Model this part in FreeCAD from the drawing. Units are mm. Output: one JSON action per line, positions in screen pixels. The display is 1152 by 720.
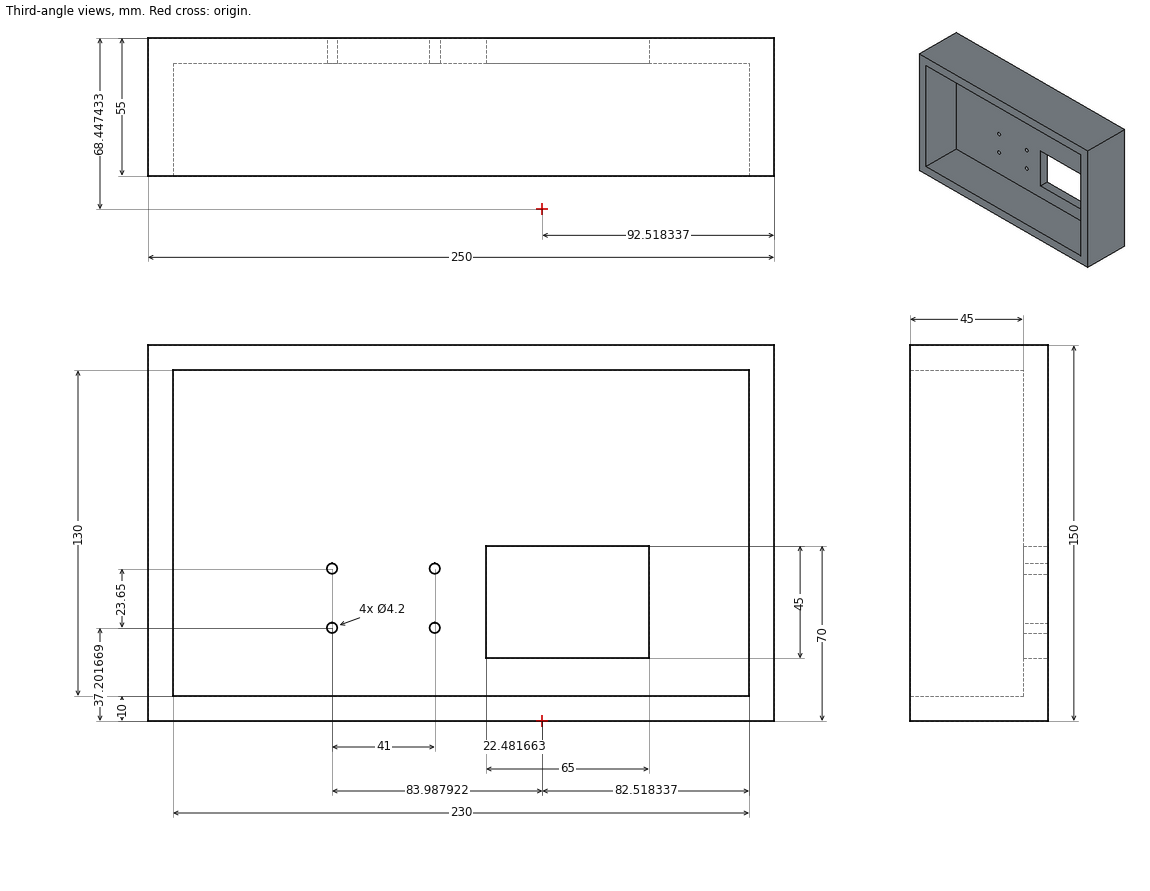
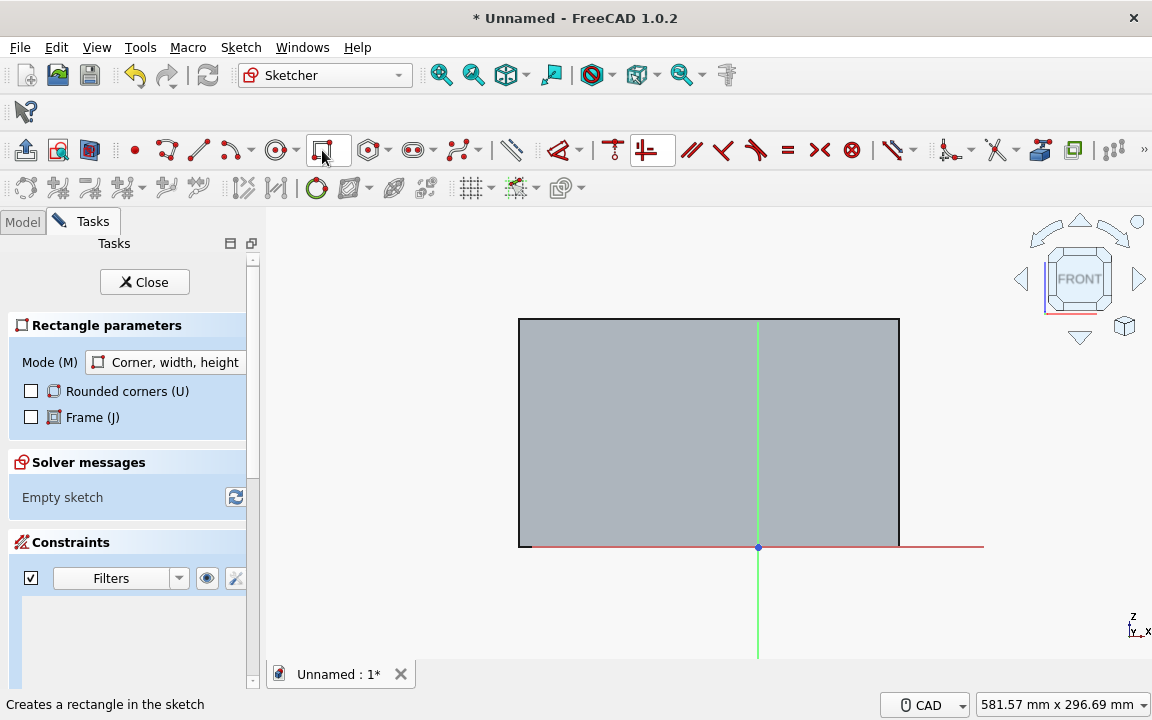
{"action": "left_click", "coordinate": [534, 334]}
{"action": "left_click", "coordinate": [884, 532]}
{"action": "key", "text": "Escape"}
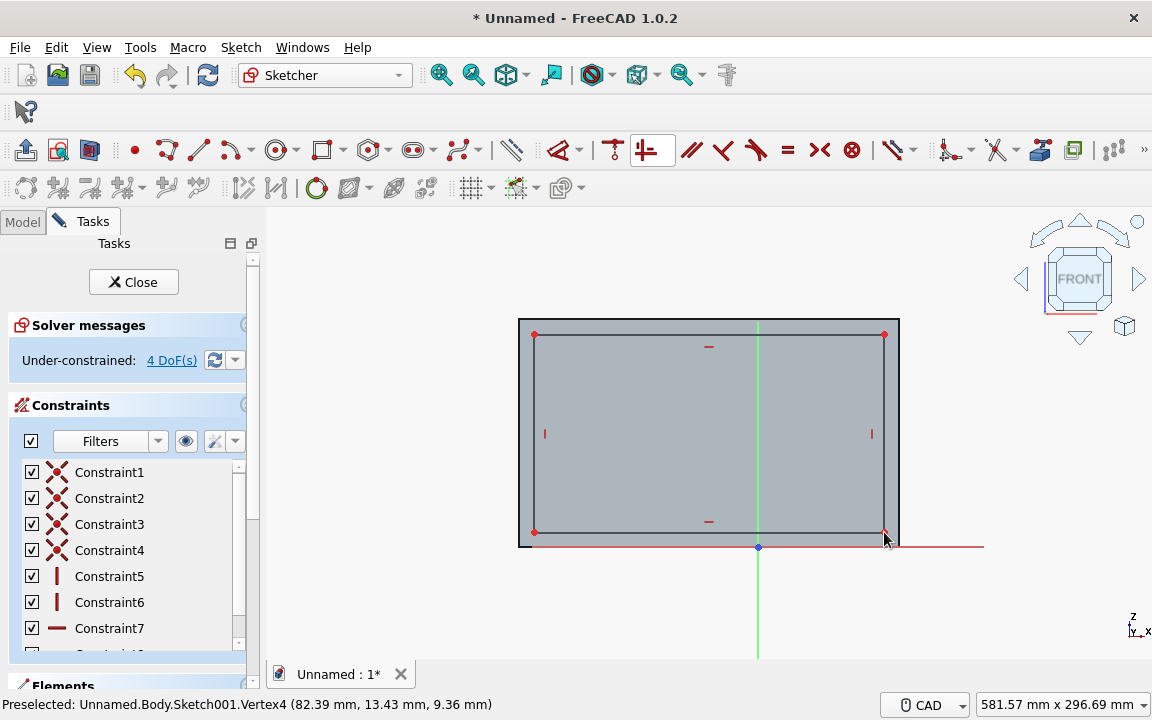
{"action": "left_click", "coordinate": [558, 150]}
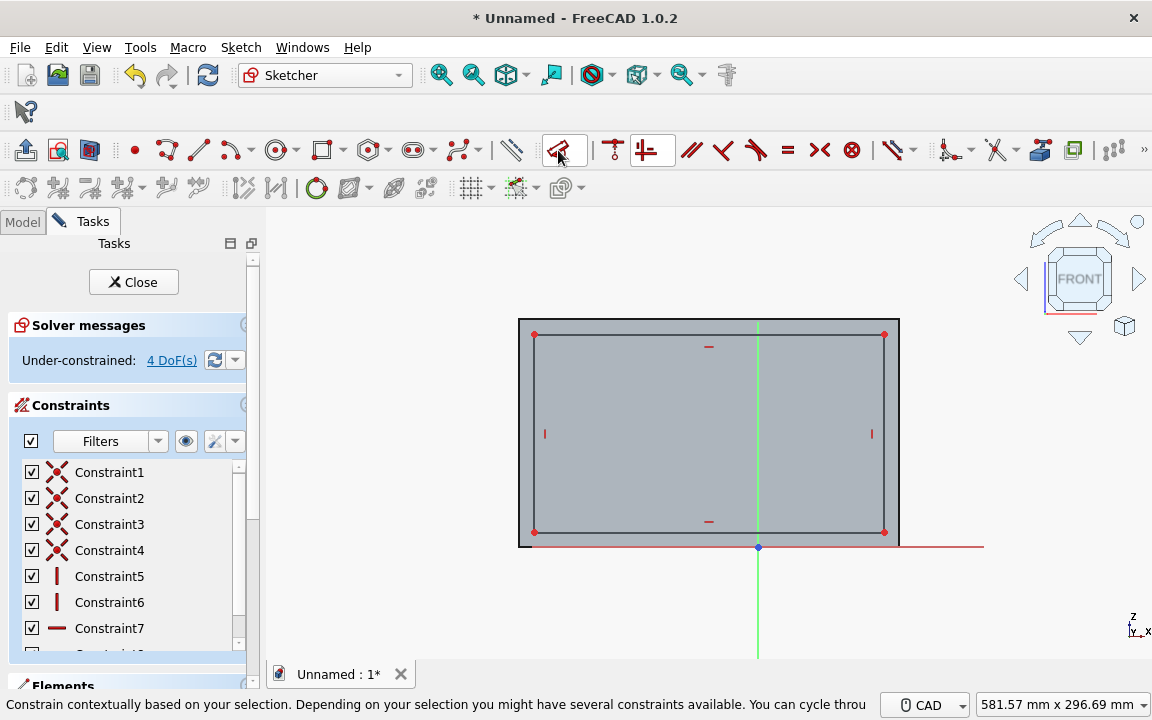
{"action": "left_click", "coordinate": [534, 394]}
{"action": "left_click", "coordinate": [500, 434]}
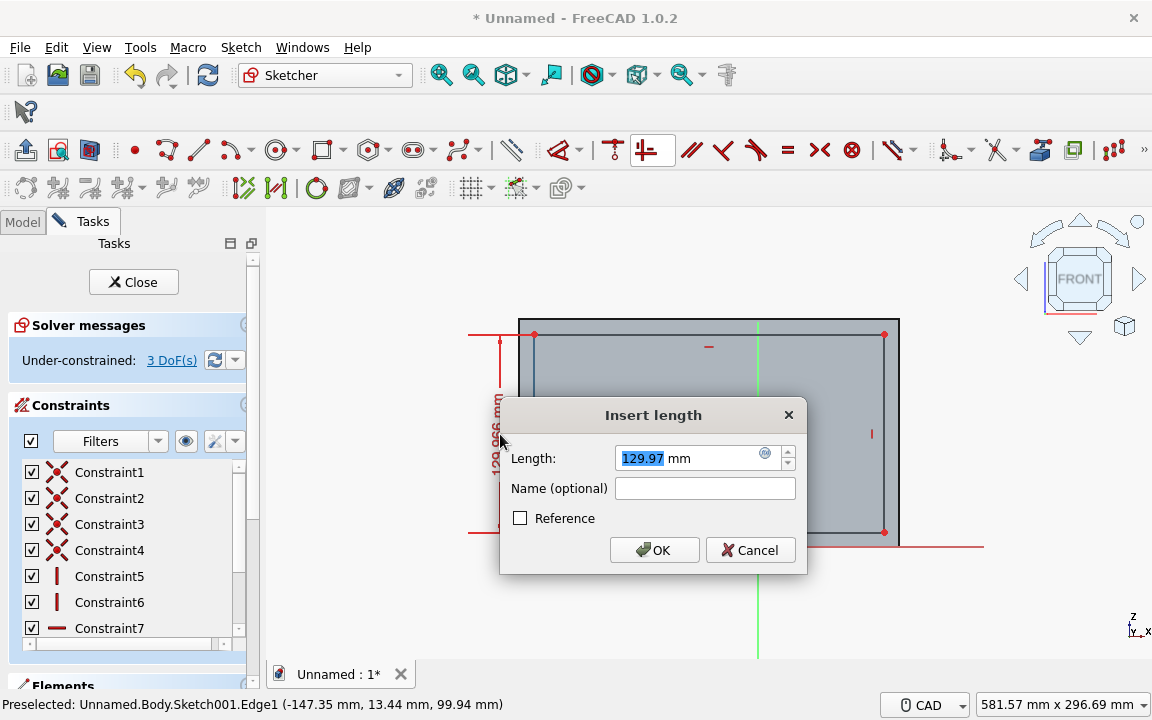
{"action": "type", "text": "130"}
{"action": "key", "text": "Return"}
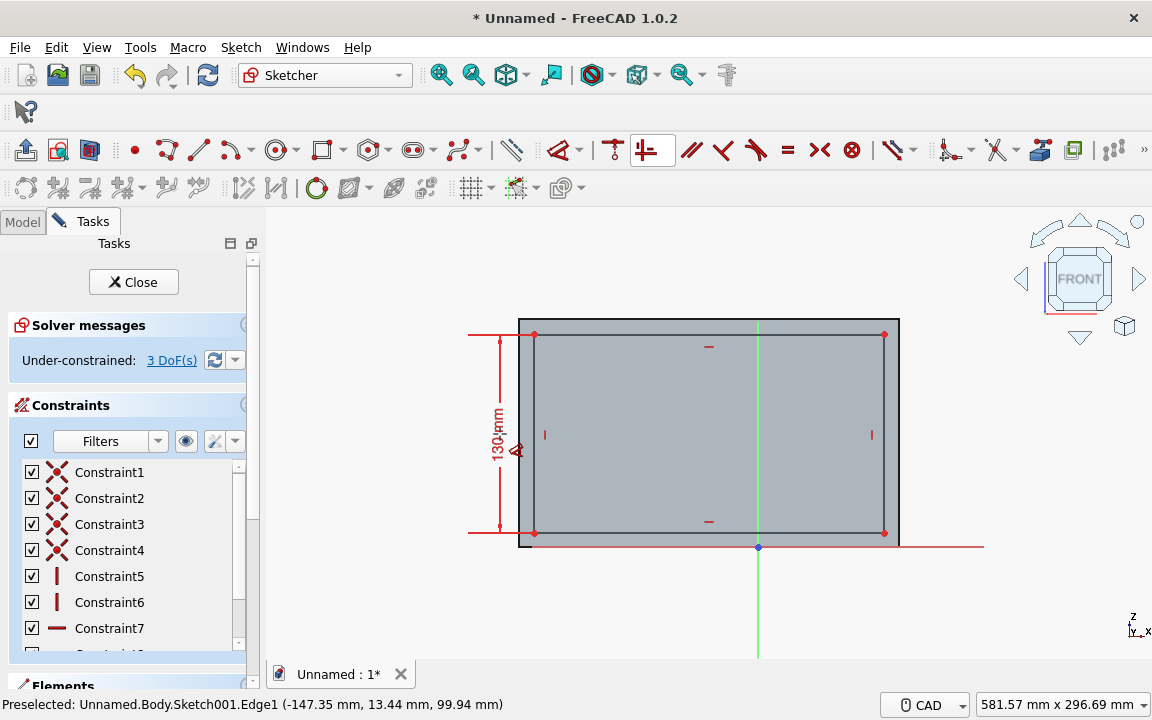
{"action": "left_click", "coordinate": [639, 533]}
{"action": "left_click", "coordinate": [709, 567]}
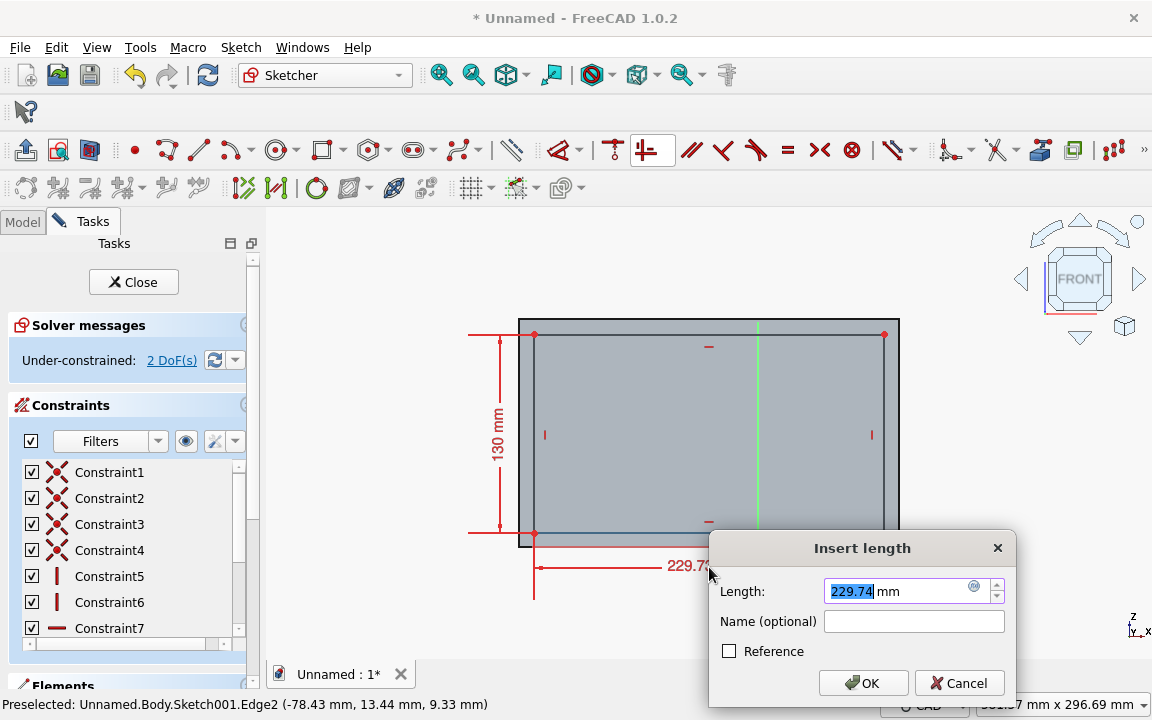
{"action": "type", "text": "230"}
{"action": "key", "text": "Return"}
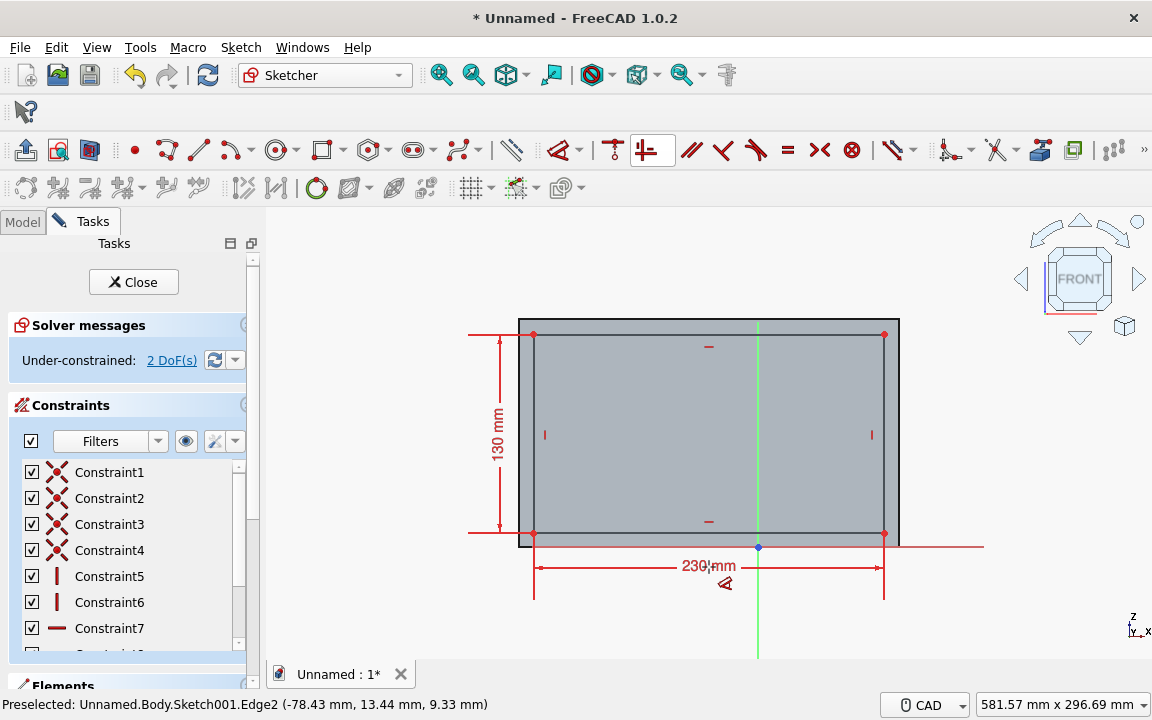
{"action": "scroll", "coordinate": [534, 533], "scroll_direction": "up", "scroll_amount": 5}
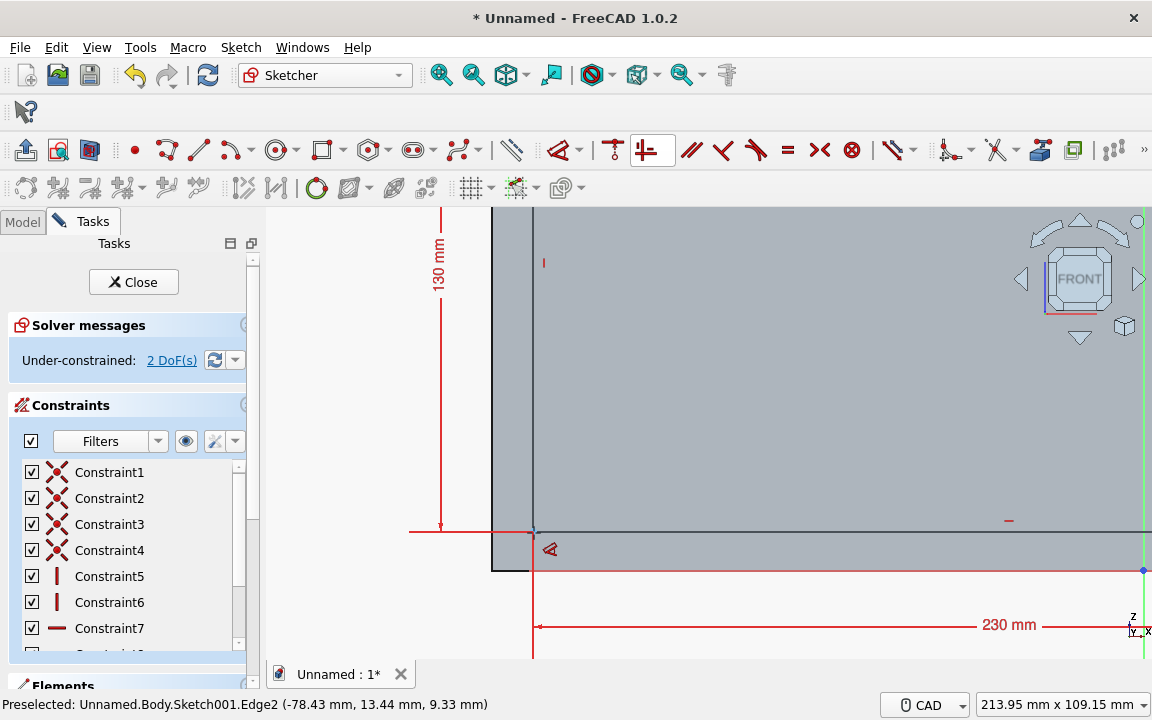
{"action": "left_click", "coordinate": [533, 532]}
{"action": "left_click", "coordinate": [499, 551]}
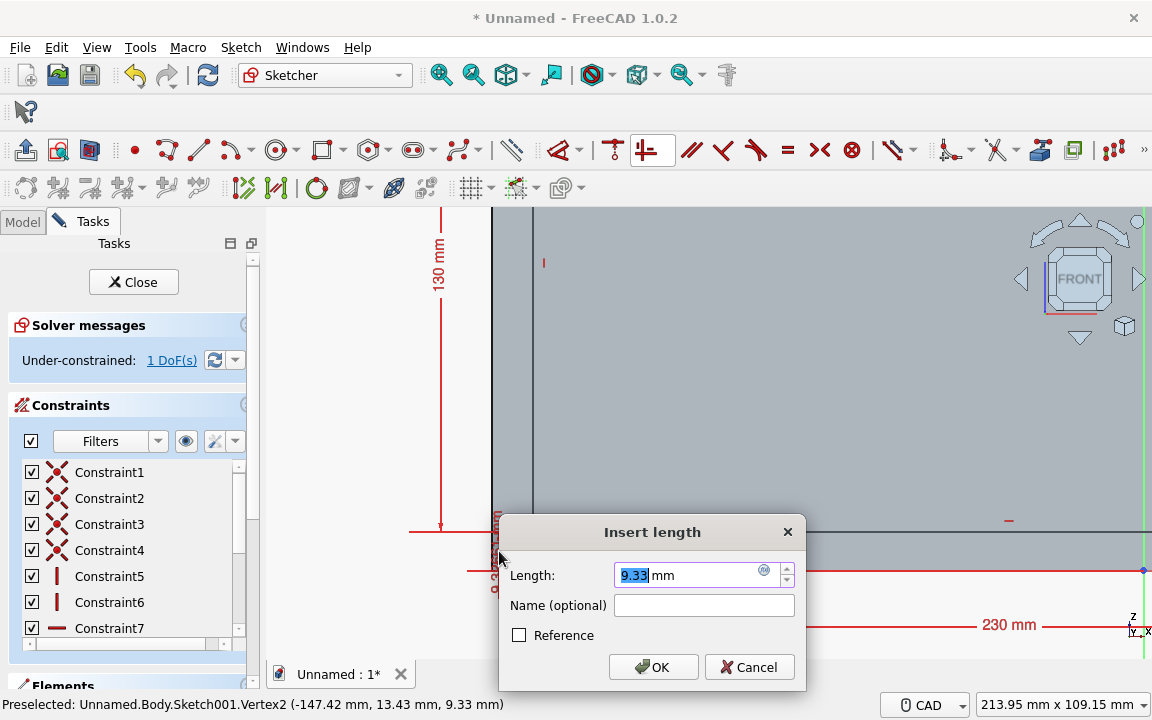
{"action": "type", "text": "10"}
{"action": "key", "text": "Return"}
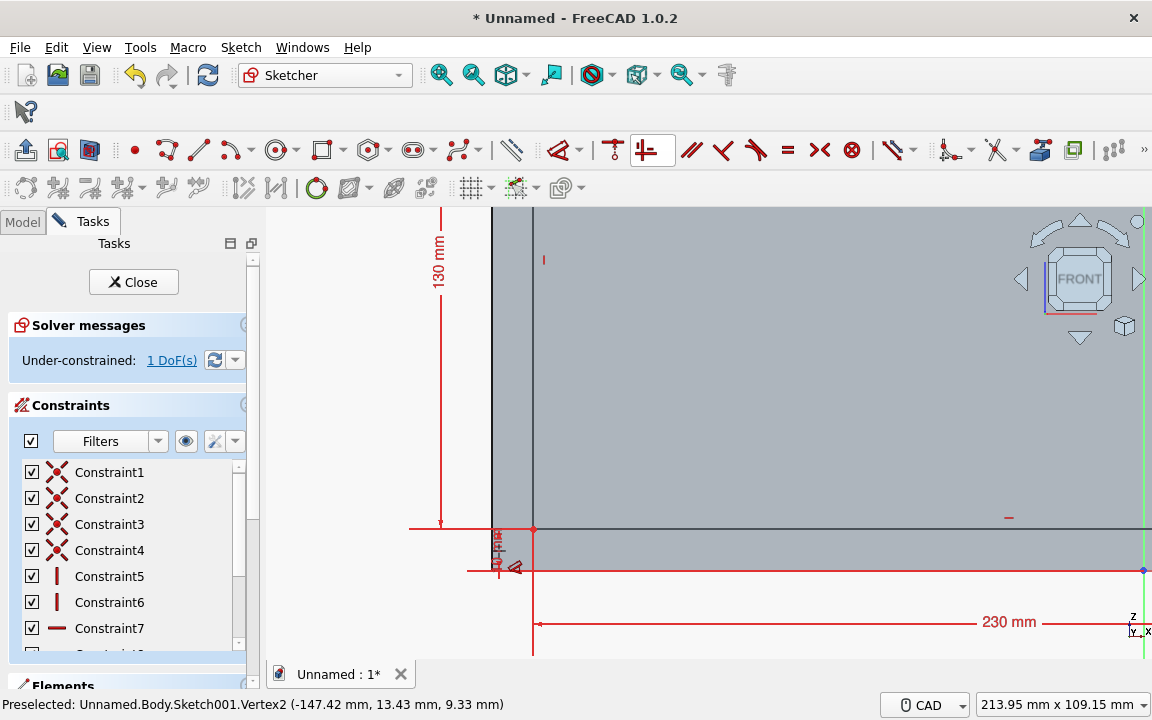
{"action": "scroll", "coordinate": [340, 557], "scroll_direction": "down", "scroll_amount": 4}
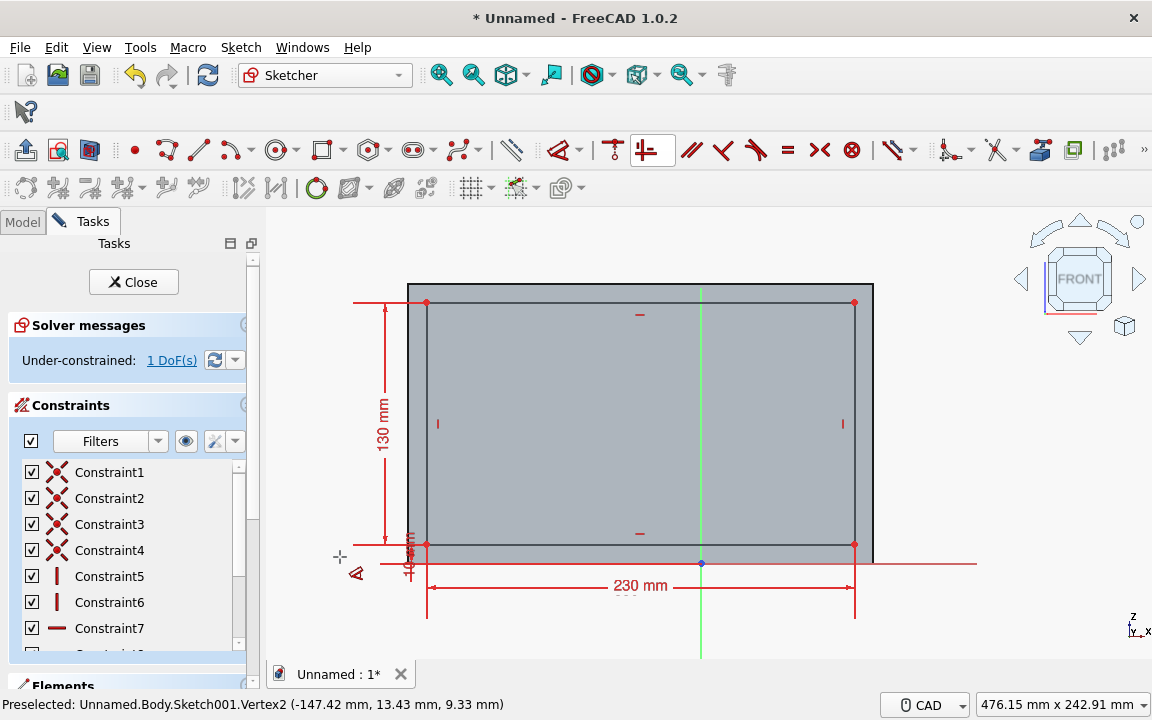
{"action": "left_click", "coordinate": [855, 545]}
{"action": "left_click", "coordinate": [778, 598]}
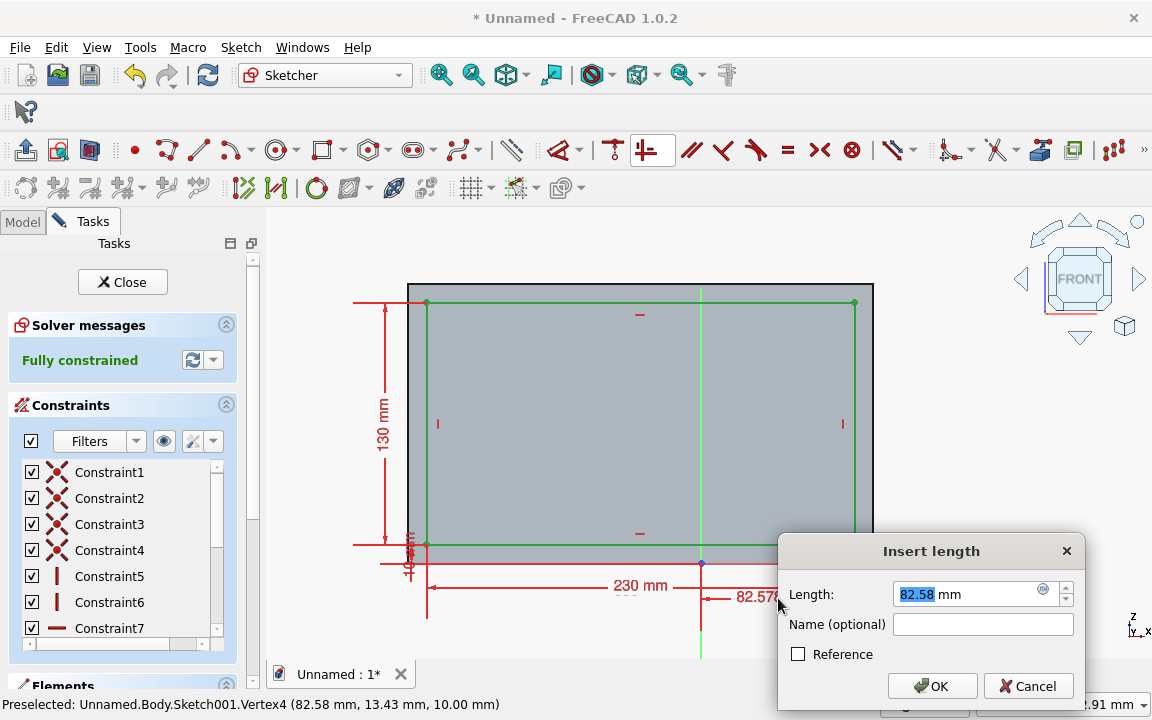
{"action": "type", "text": "82.518337"}
{"action": "key", "text": "Return"}
{"action": "key", "text": "Escape"}